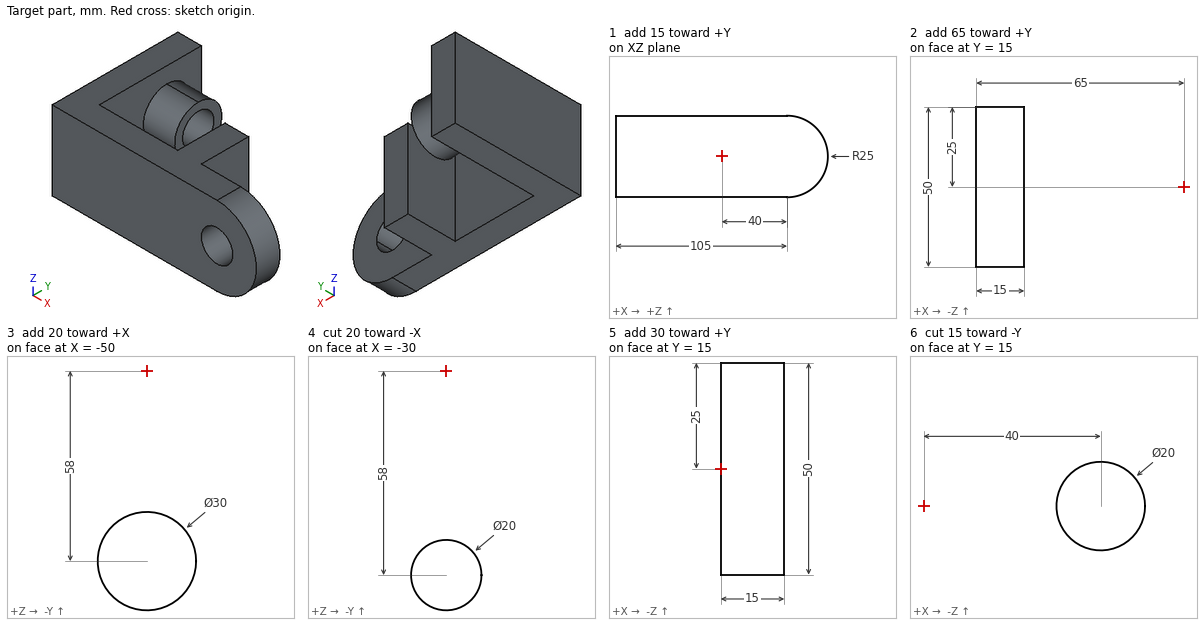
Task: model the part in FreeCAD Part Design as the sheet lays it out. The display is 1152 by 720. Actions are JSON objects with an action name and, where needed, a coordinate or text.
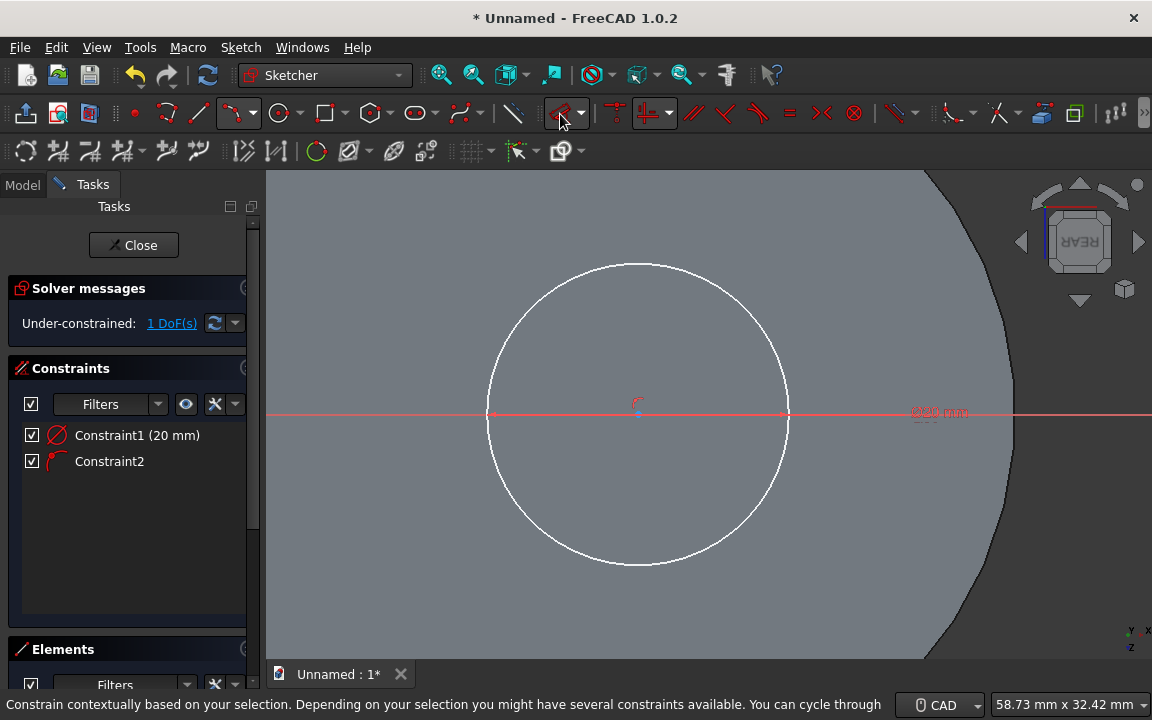
{"action": "left_click", "coordinate": [638, 414]}
{"action": "left_click", "coordinate": [466, 448]}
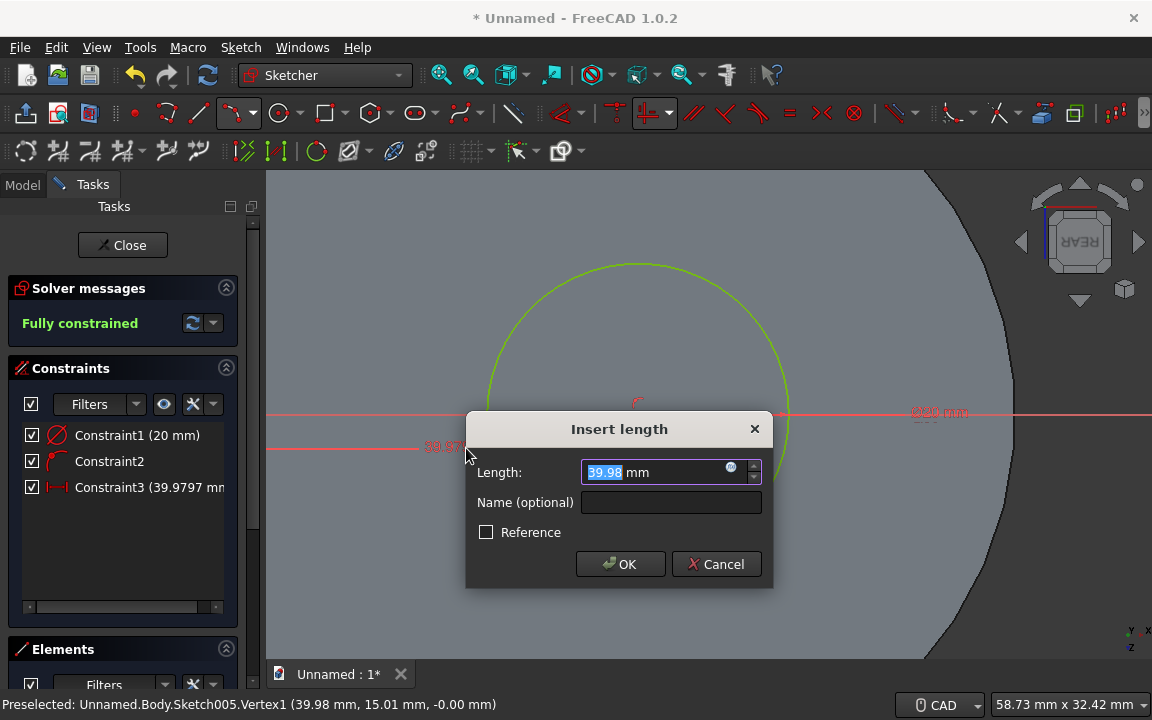
{"action": "type", "text": "40"}
{"action": "key", "text": "Return"}
{"action": "key", "text": "Escape"}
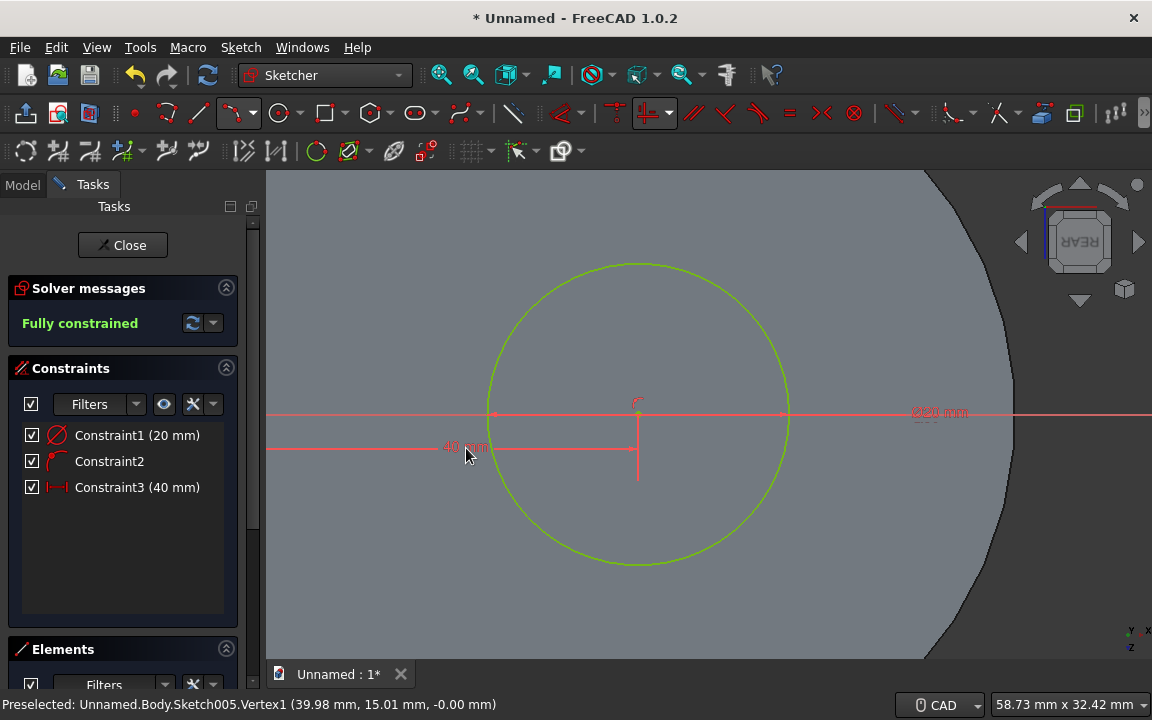
{"action": "left_click", "coordinate": [123, 245]}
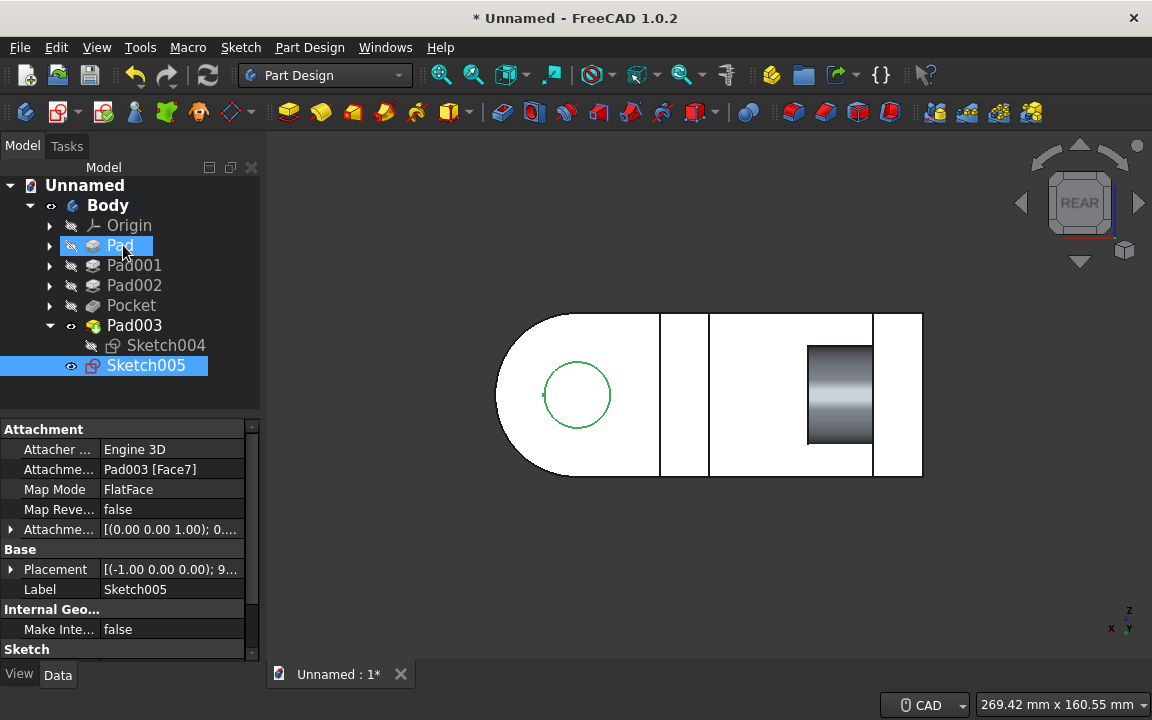
{"action": "left_click", "coordinate": [504, 112]}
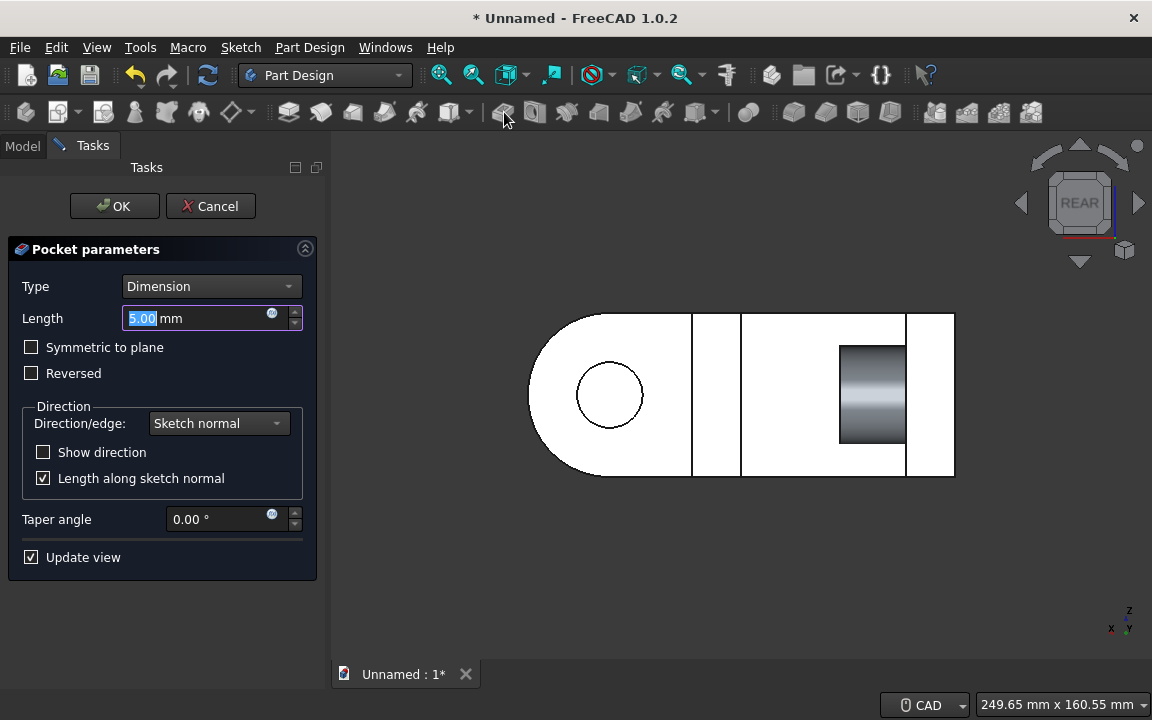
{"action": "type", "text": "15"}
{"action": "key", "text": "Tab"}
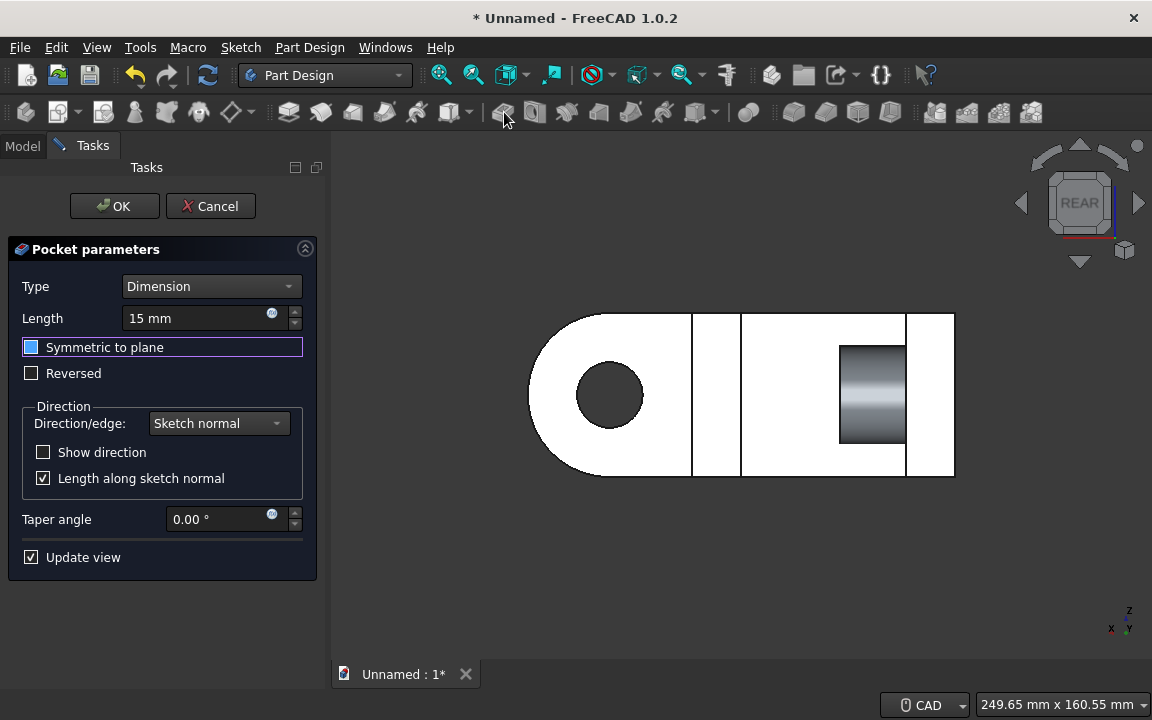
{"action": "left_click", "coordinate": [115, 206]}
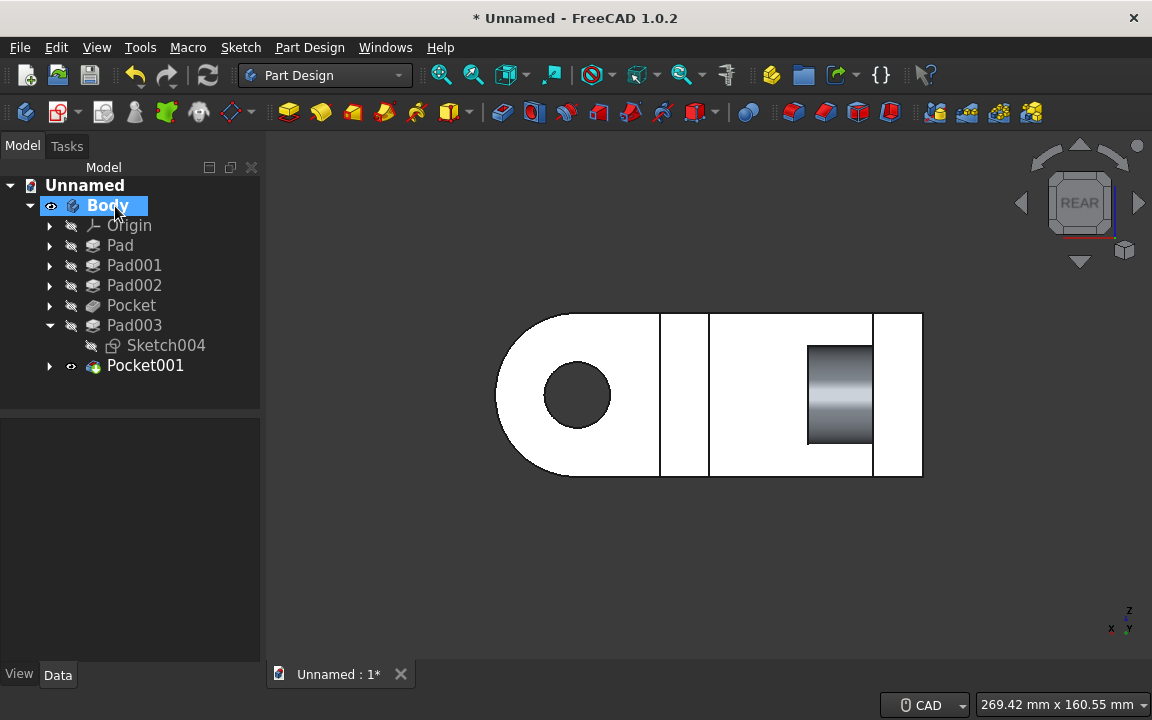
{"action": "key", "text": "0"}